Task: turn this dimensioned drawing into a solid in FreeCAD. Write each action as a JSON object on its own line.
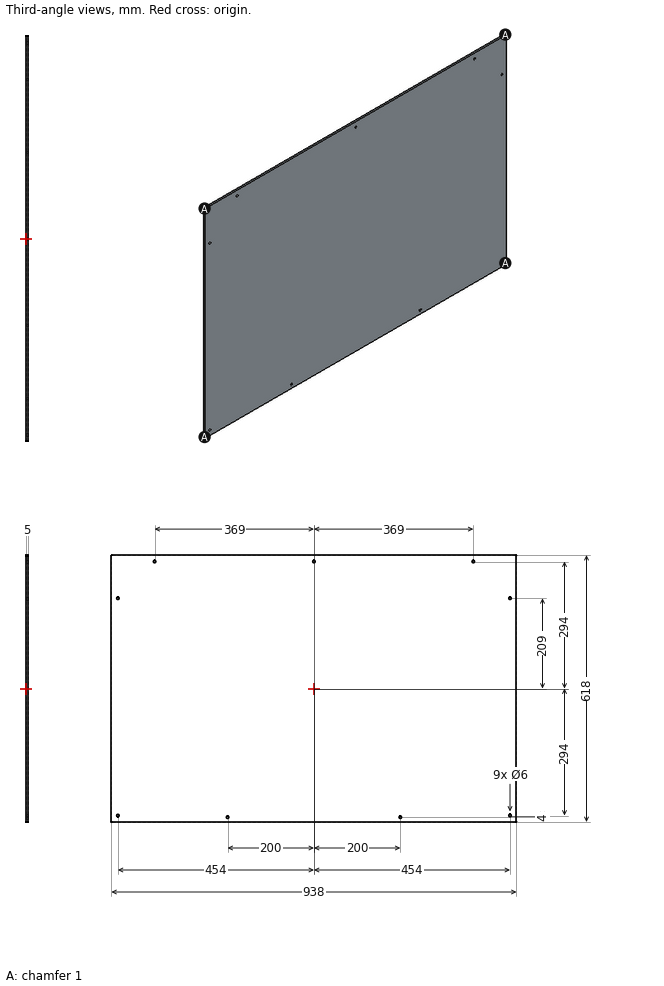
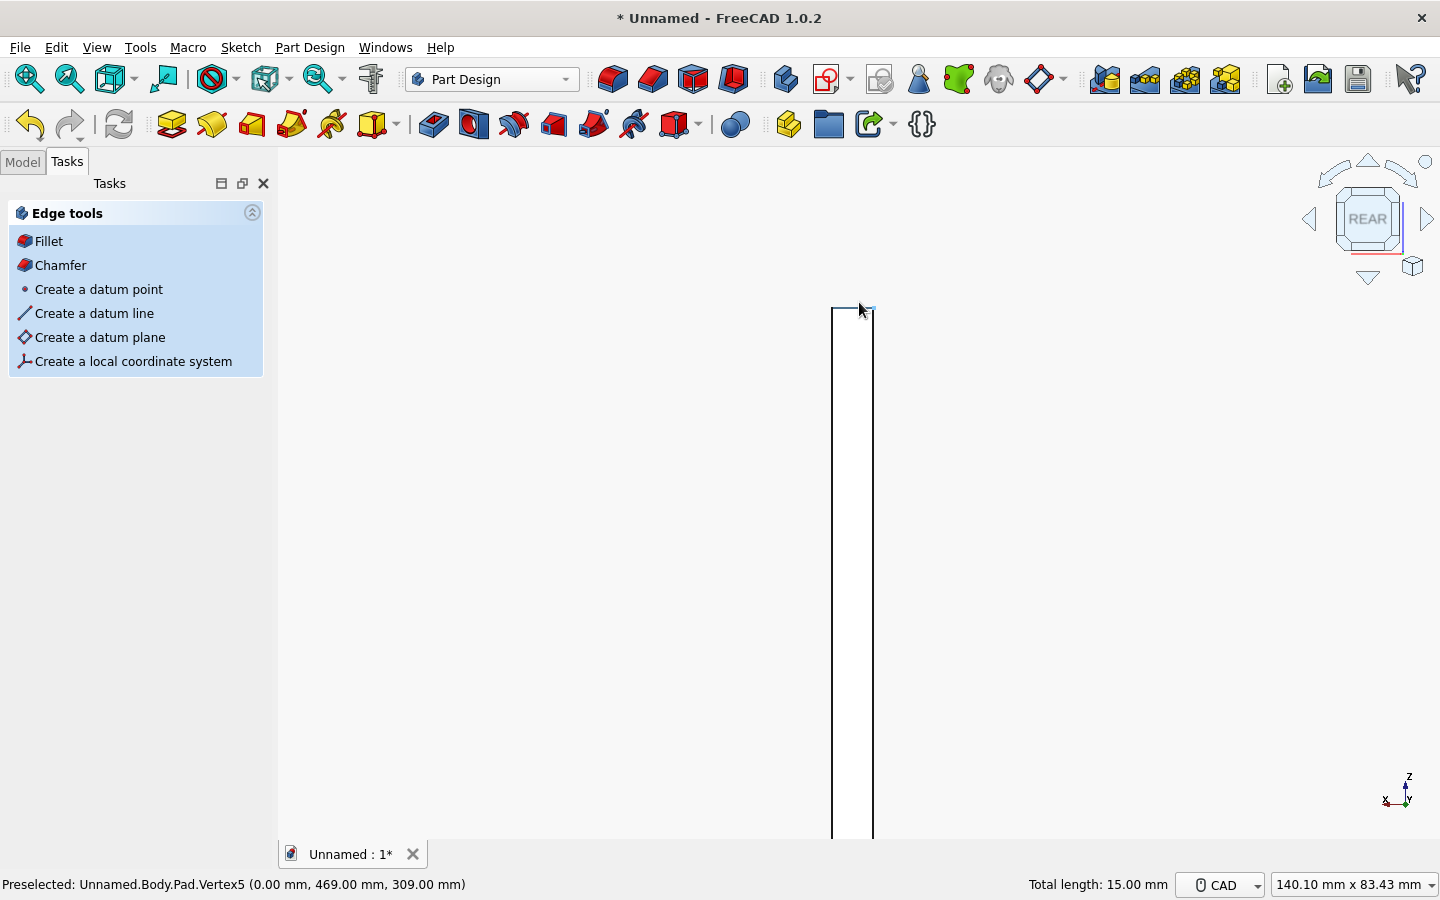
{"action": "left_click", "coordinate": [30, 80]}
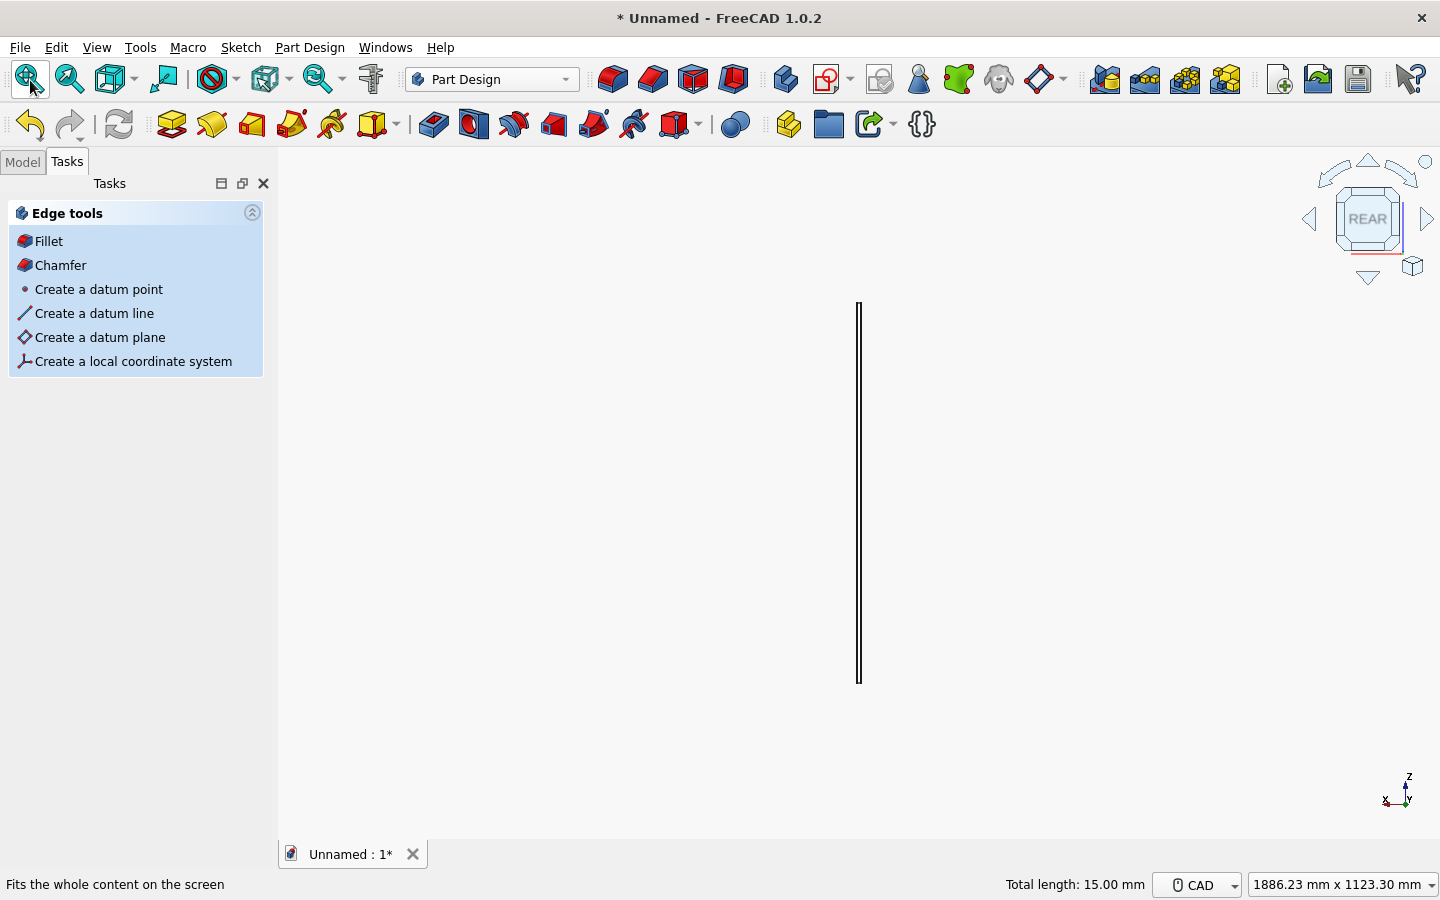
{"action": "key", "text": "6"}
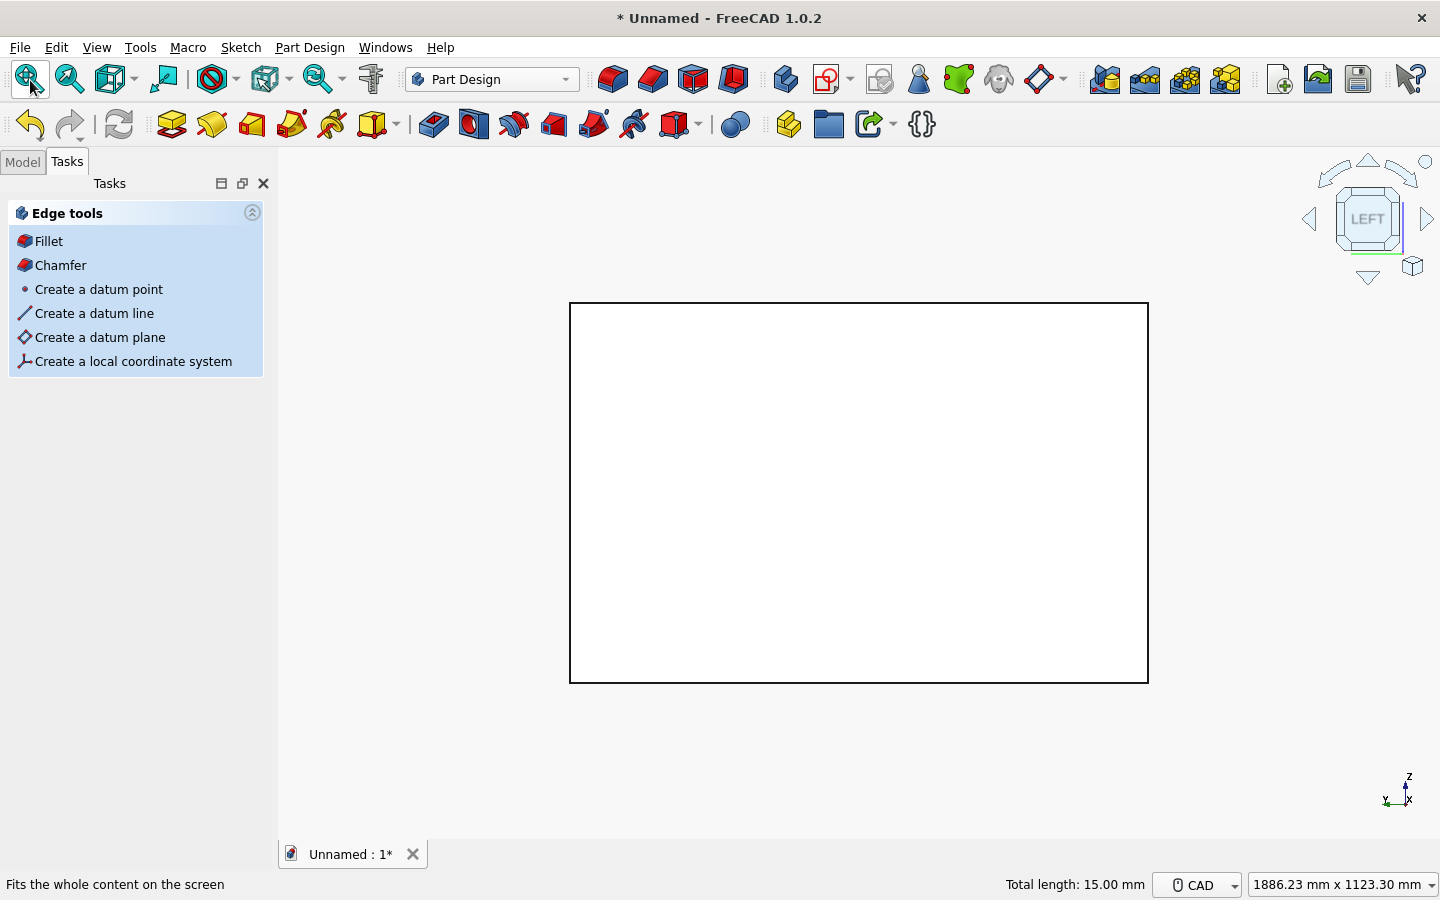
{"action": "scroll", "coordinate": [1148, 302], "scroll_direction": "up", "scroll_amount": 13}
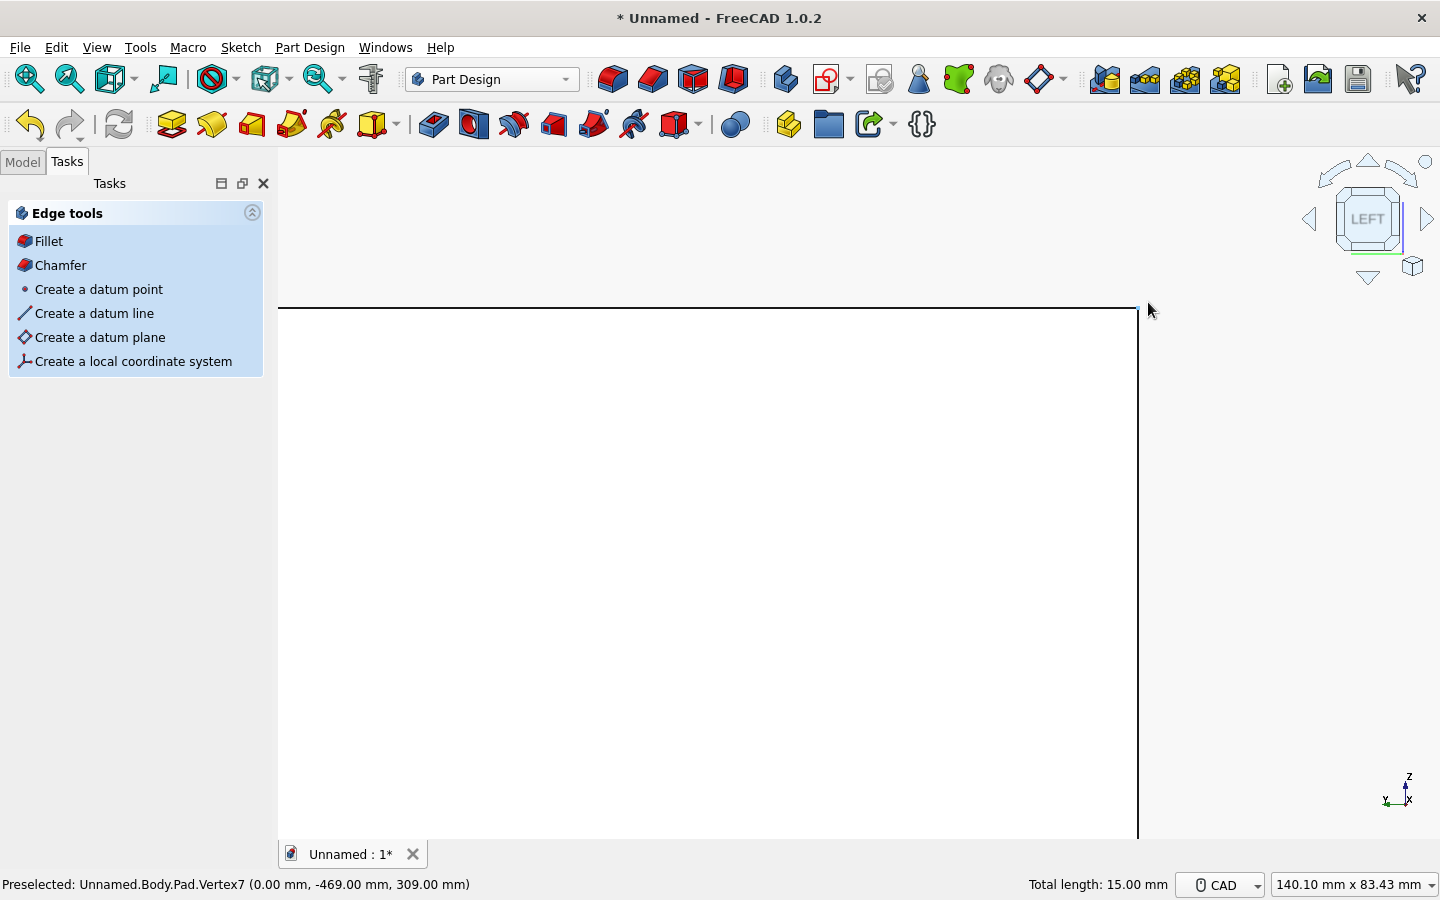
{"action": "left_click", "coordinate": [30, 80]}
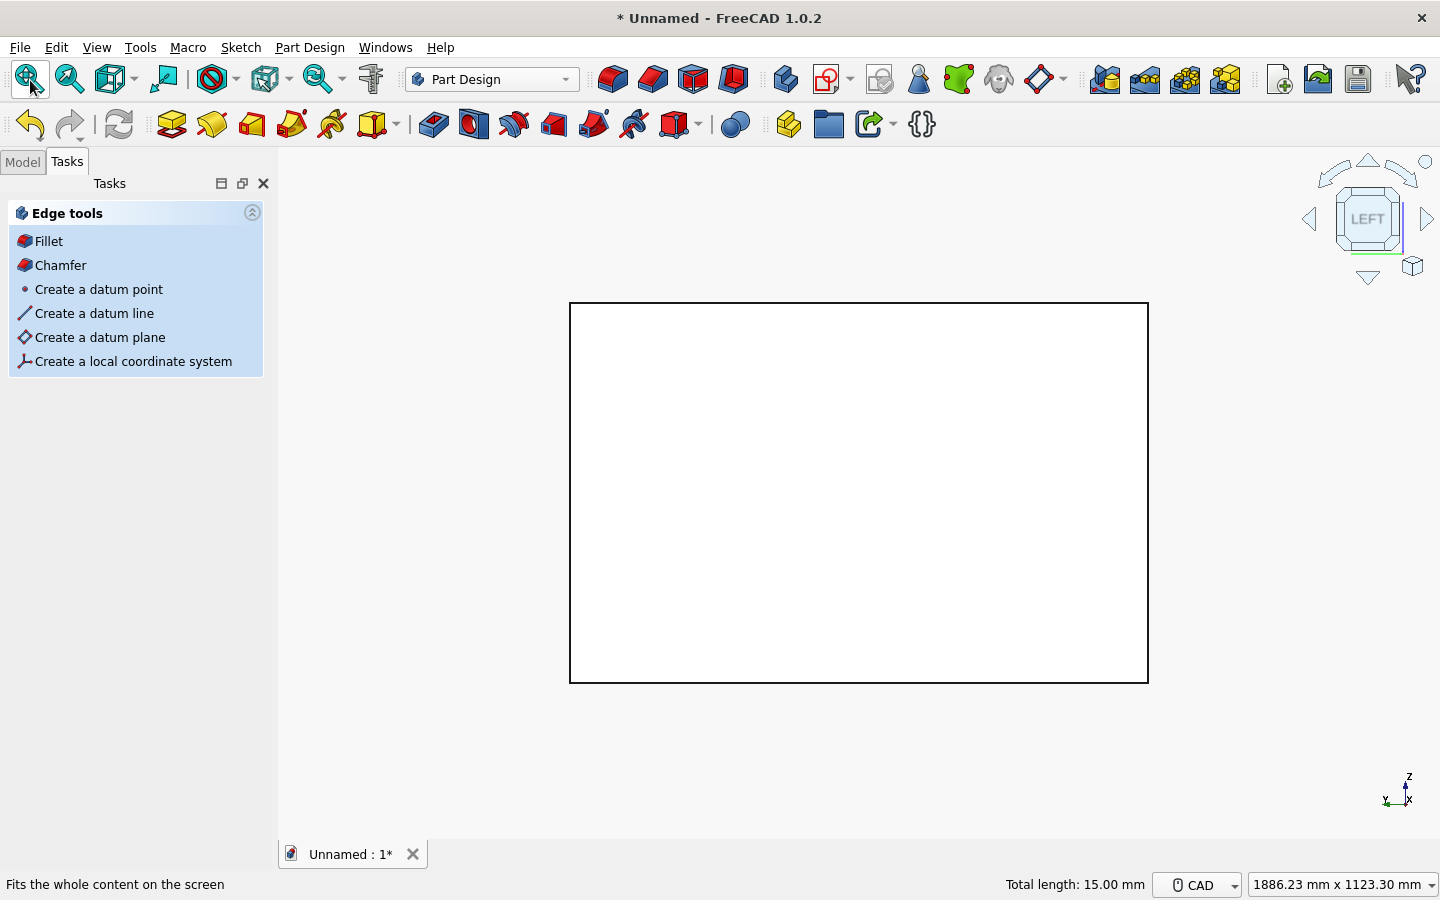
{"action": "key", "text": "v 3"}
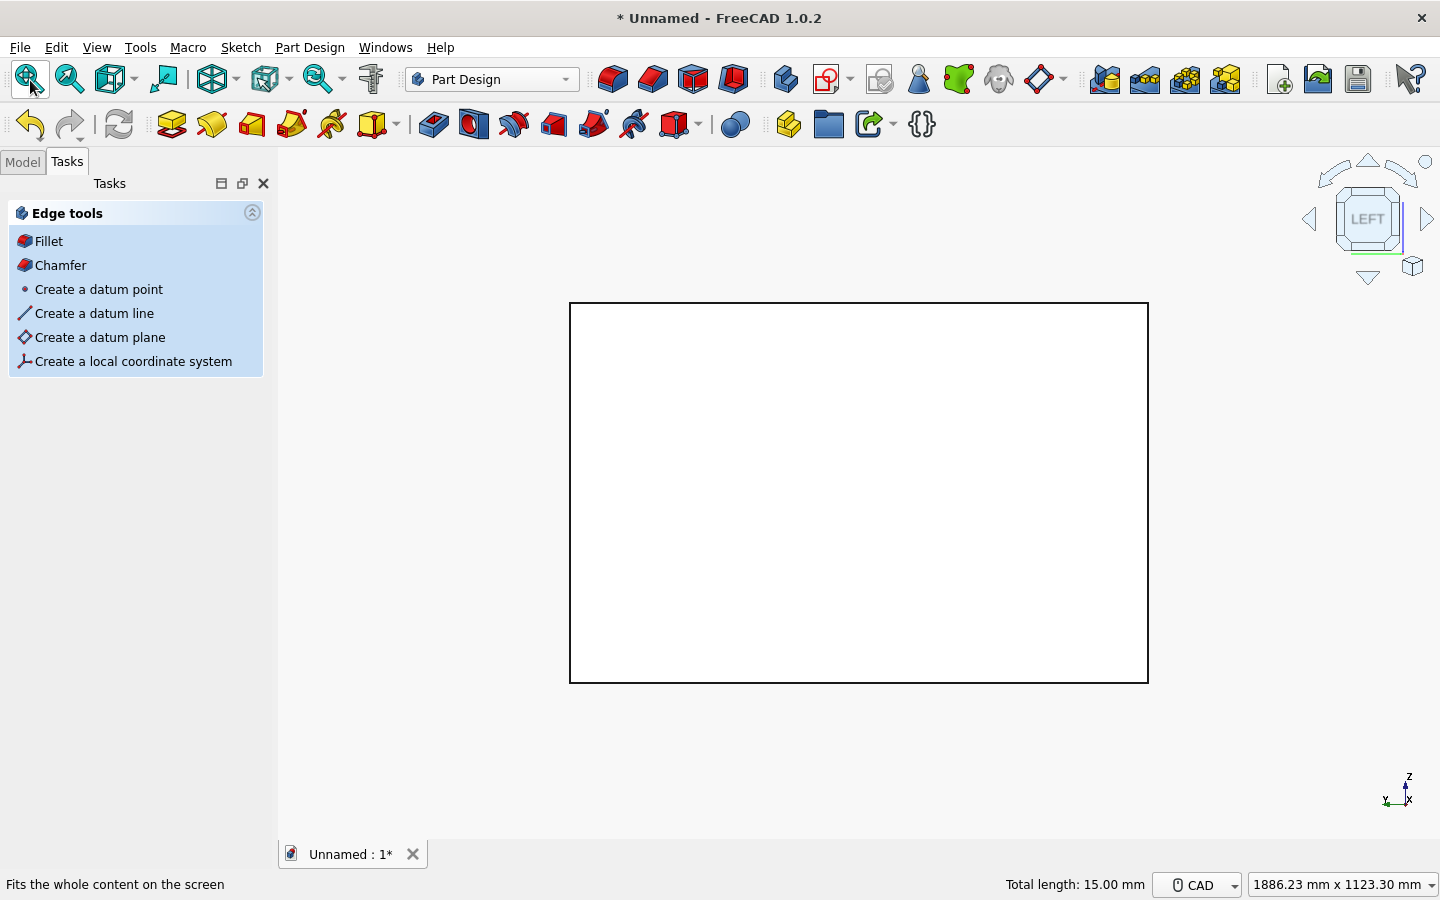
{"action": "key", "text": "0"}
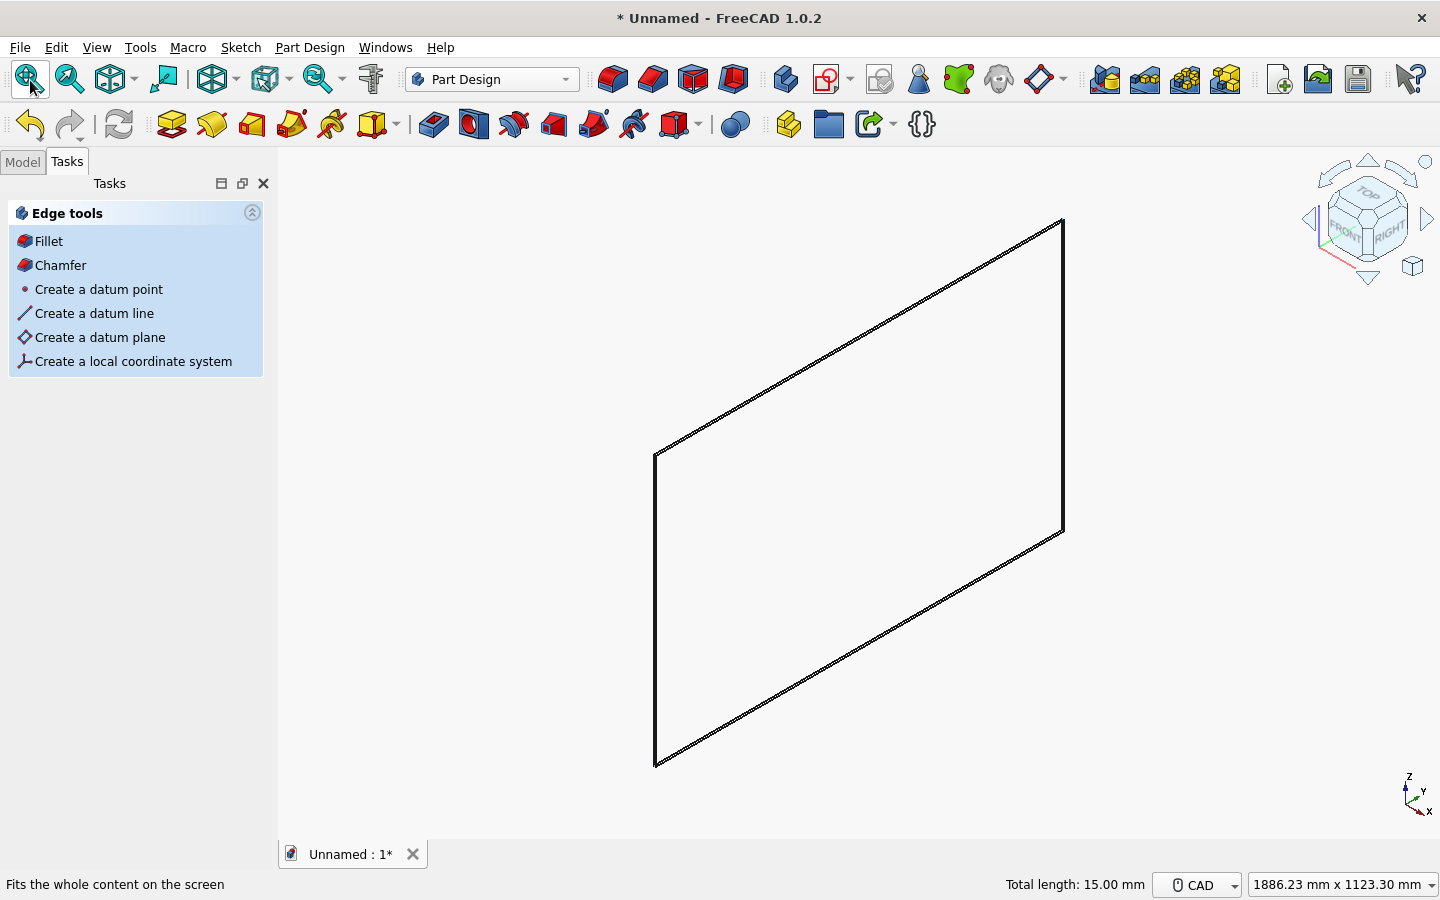
{"action": "scroll", "coordinate": [655, 455], "scroll_direction": "up", "scroll_amount": 13}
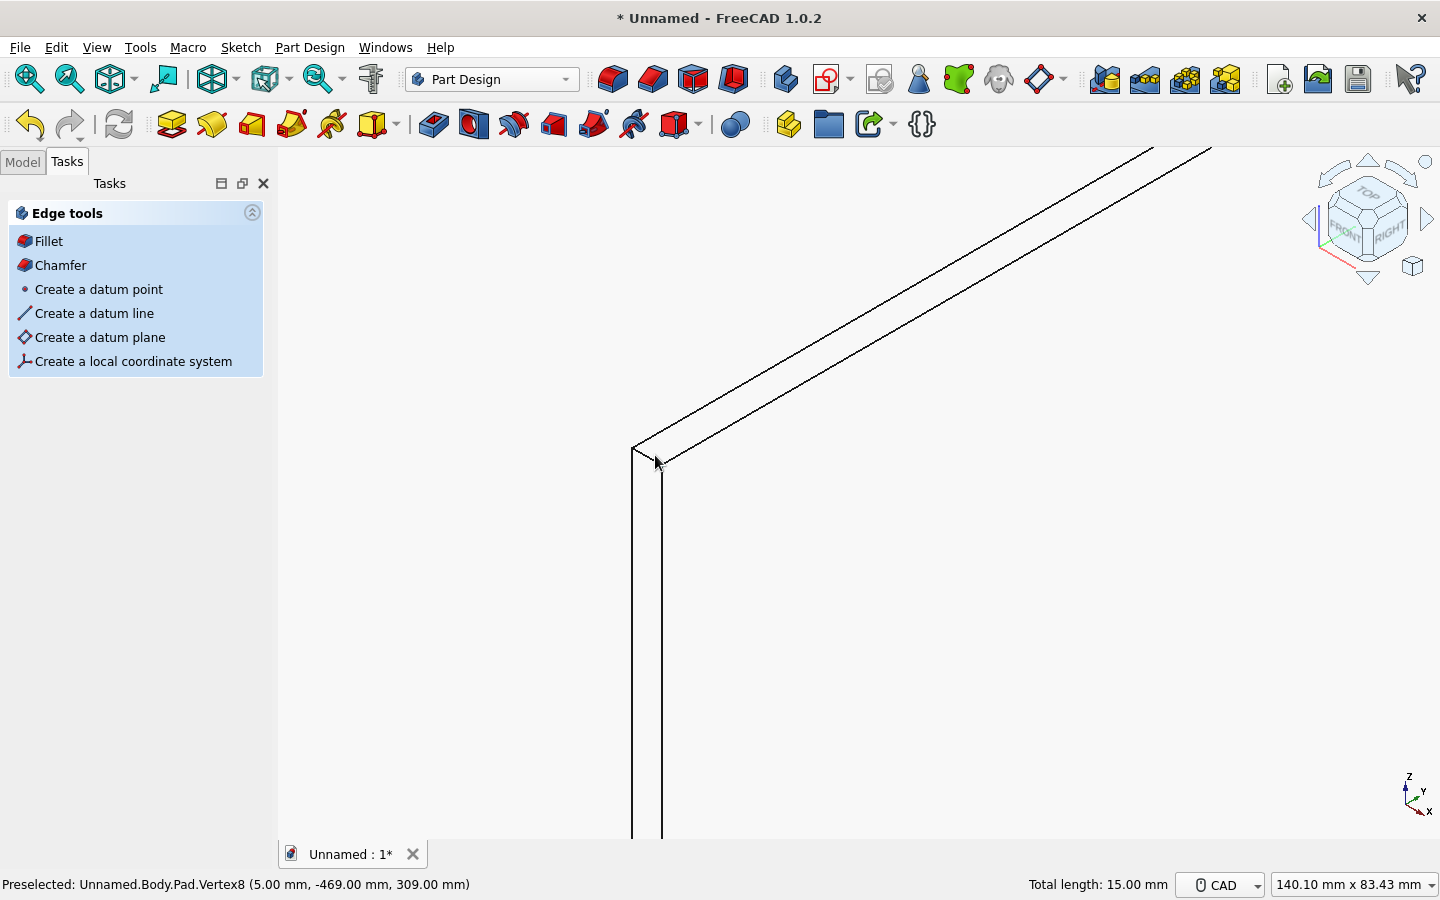
{"action": "left_click", "coordinate": [647, 456], "text": "ctrl"}